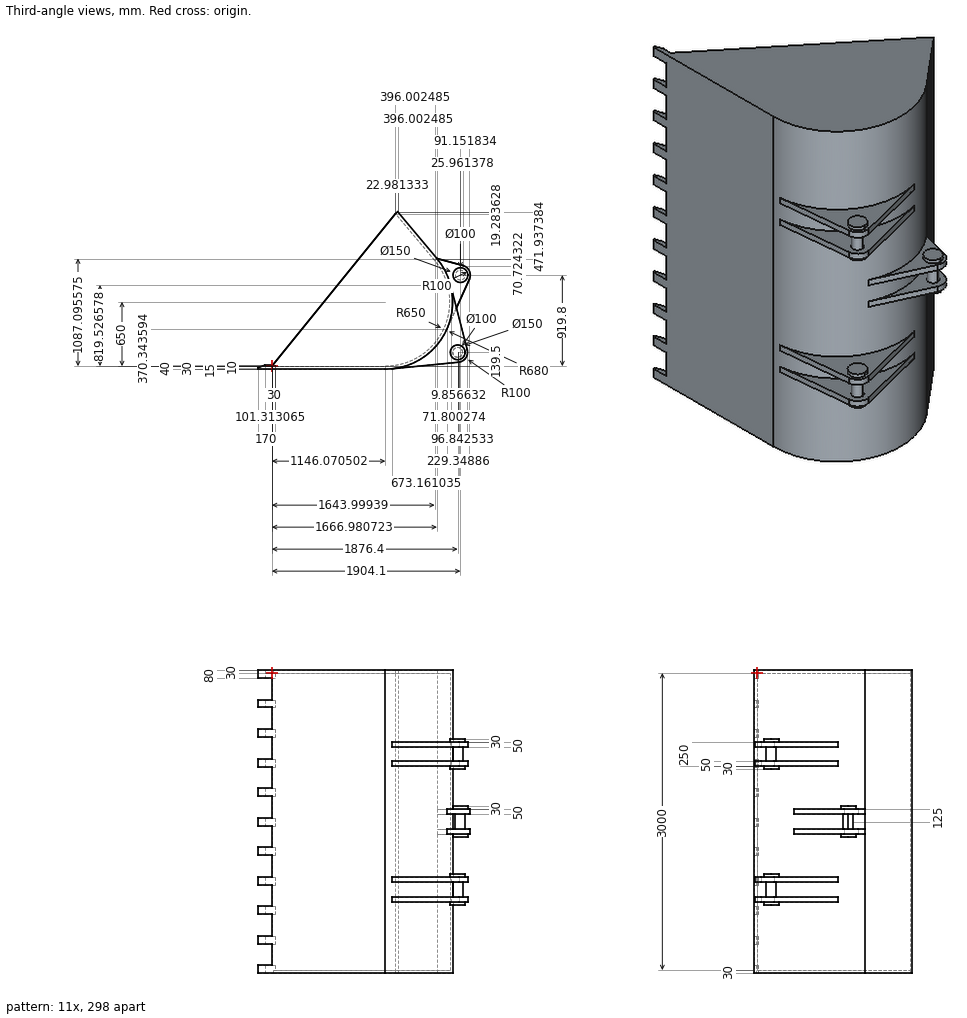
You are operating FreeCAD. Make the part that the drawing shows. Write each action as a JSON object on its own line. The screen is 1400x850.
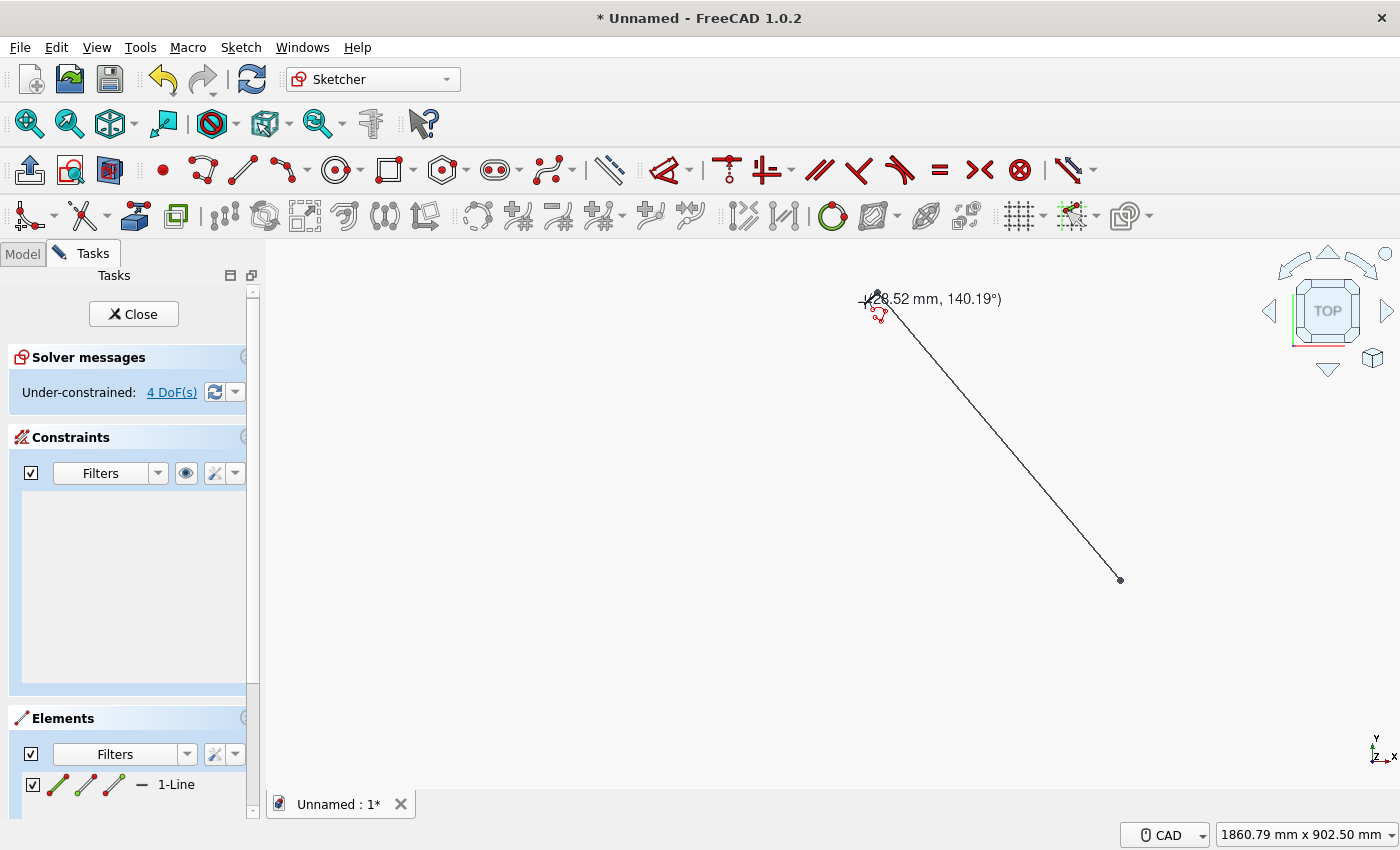
{"action": "left_click", "coordinate": [865, 302]}
{"action": "left_click", "coordinate": [1106, 590]}
{"action": "right_click", "coordinate": [1106, 590]}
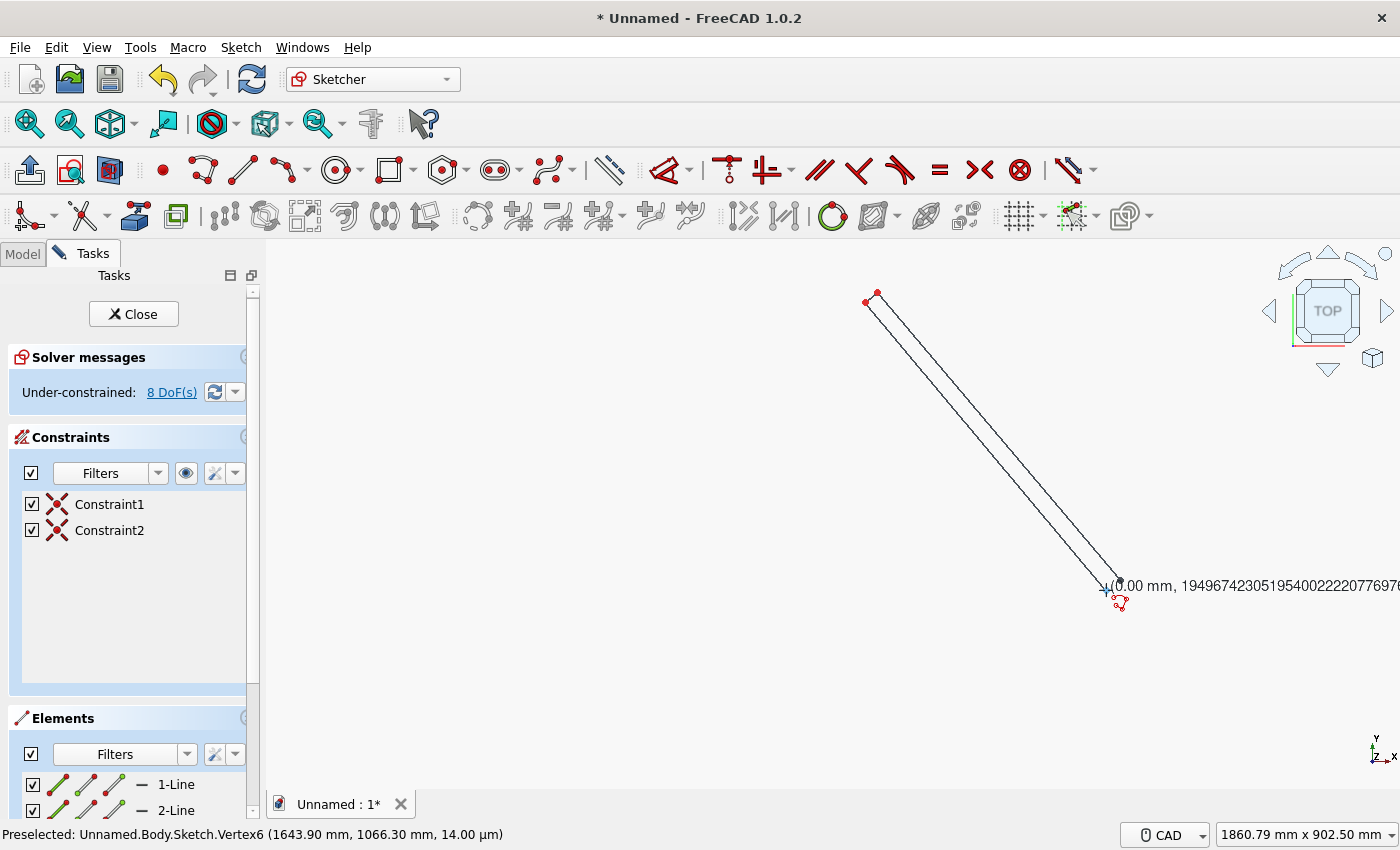
{"action": "scroll", "coordinate": [836, 362], "scroll_direction": "down", "scroll_amount": 5}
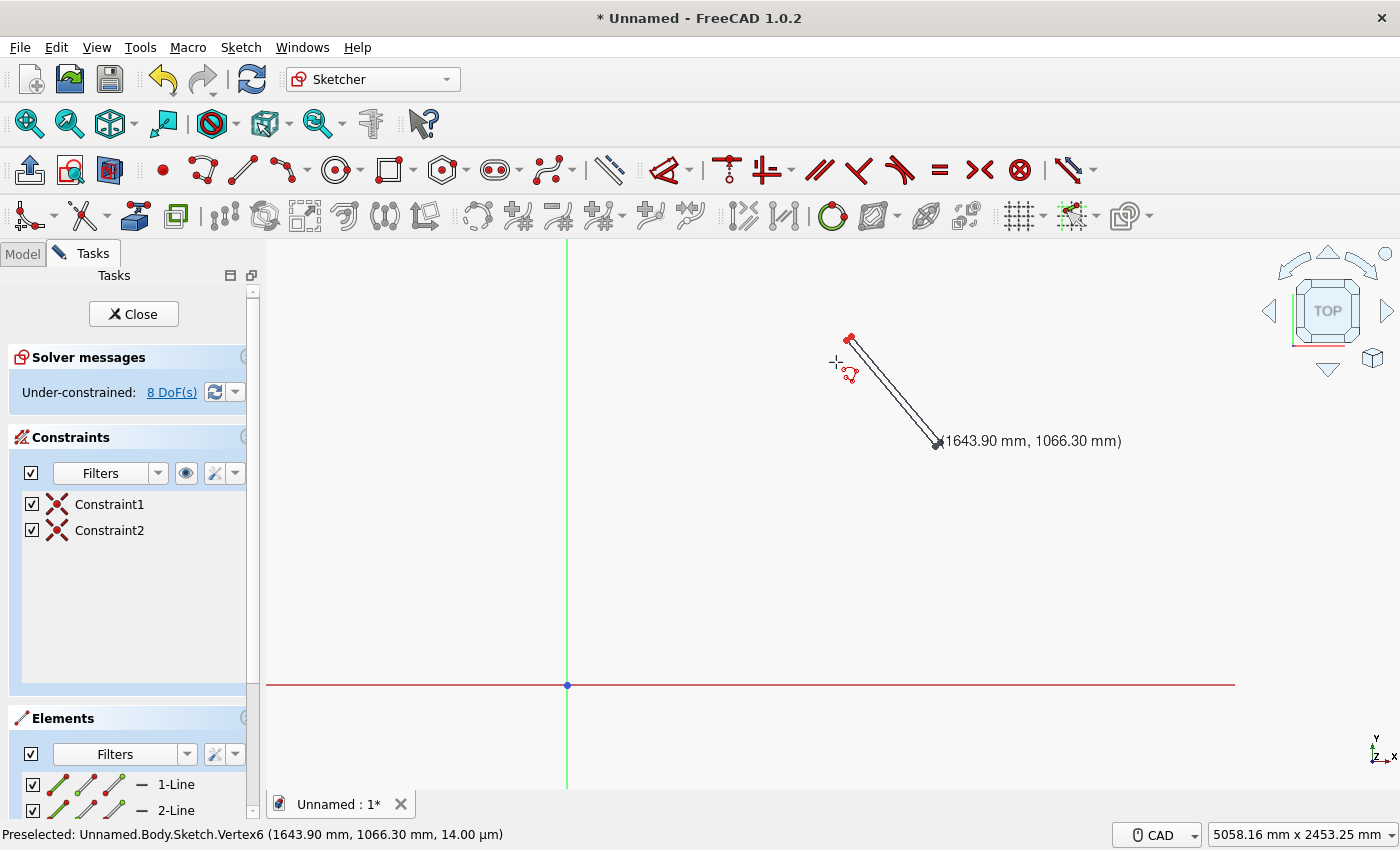
{"action": "left_click", "coordinate": [824, 685]}
{"action": "left_click", "coordinate": [567, 685]}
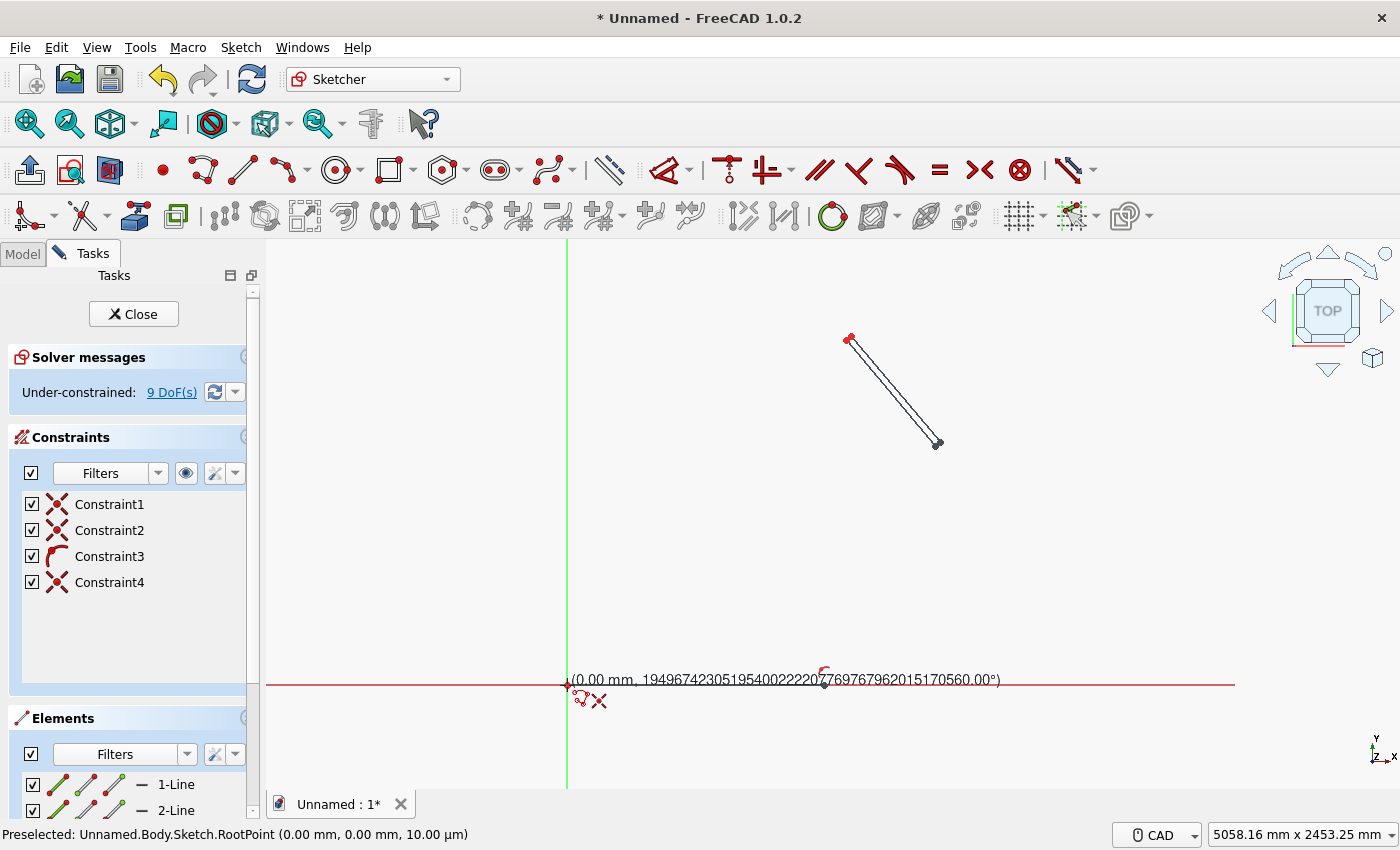
{"action": "scroll", "coordinate": [567, 692], "scroll_direction": "up", "scroll_amount": 5}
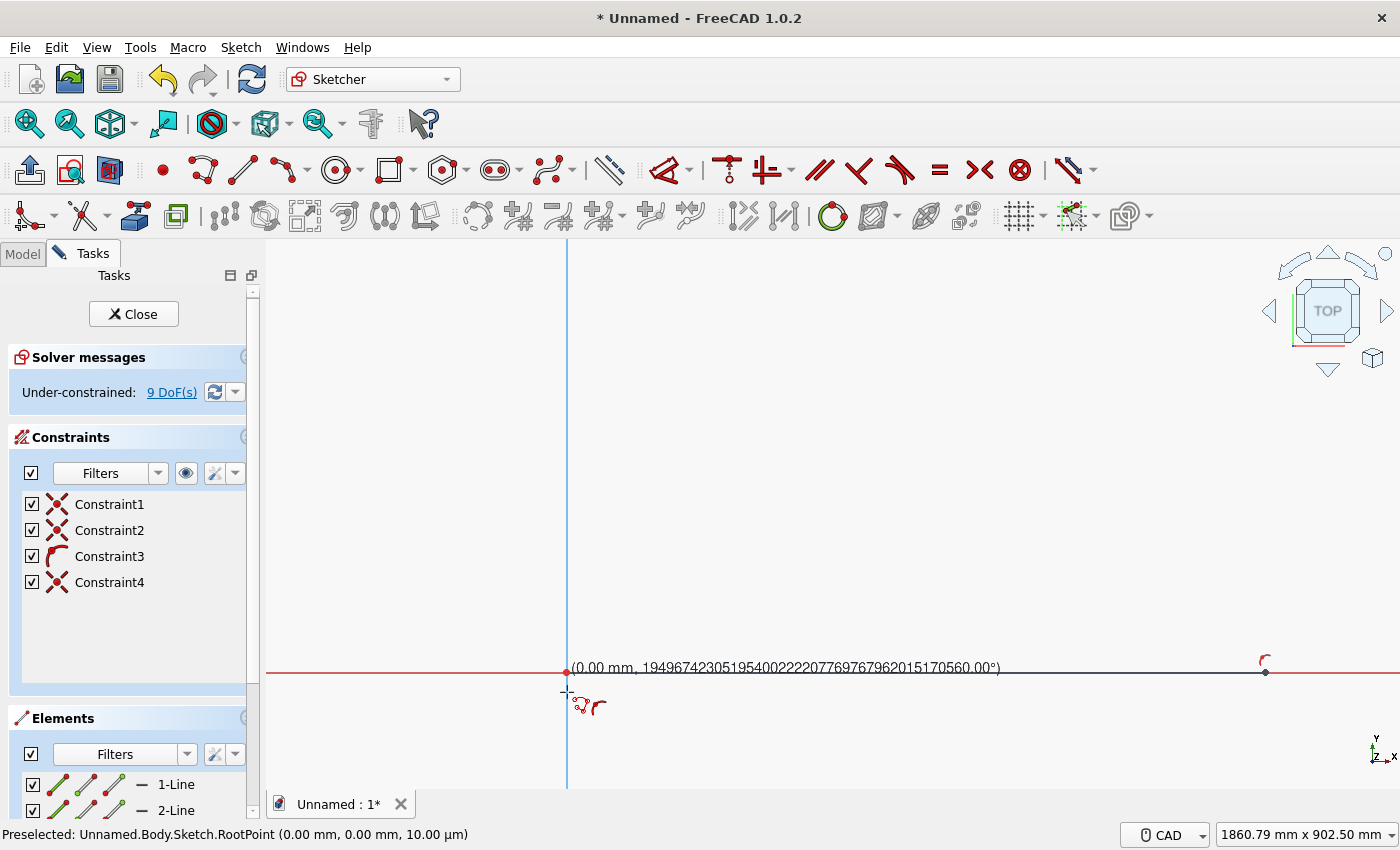
{"action": "left_click", "coordinate": [576, 691]}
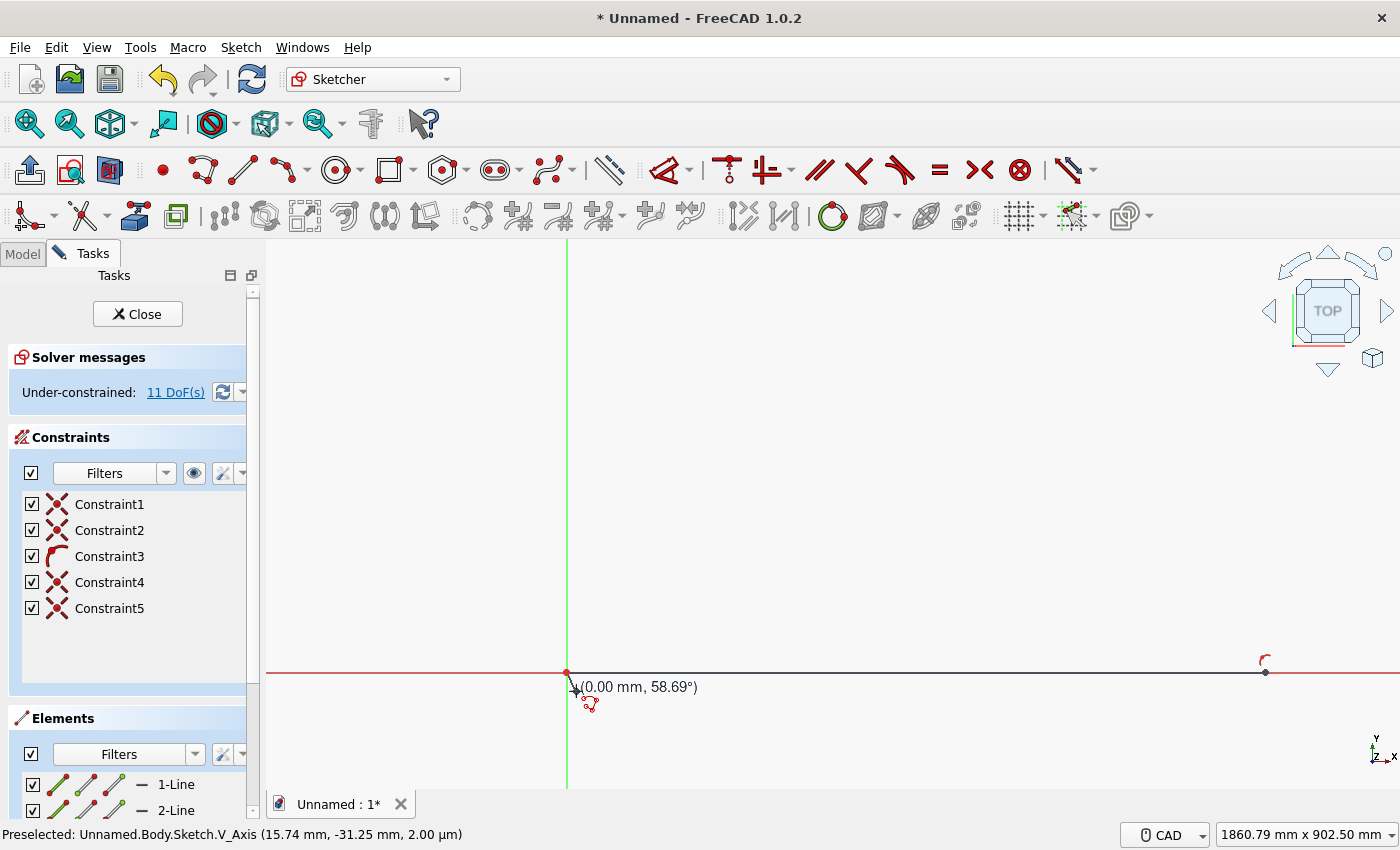
{"action": "scroll", "coordinate": [567, 693], "scroll_direction": "down", "scroll_amount": 5}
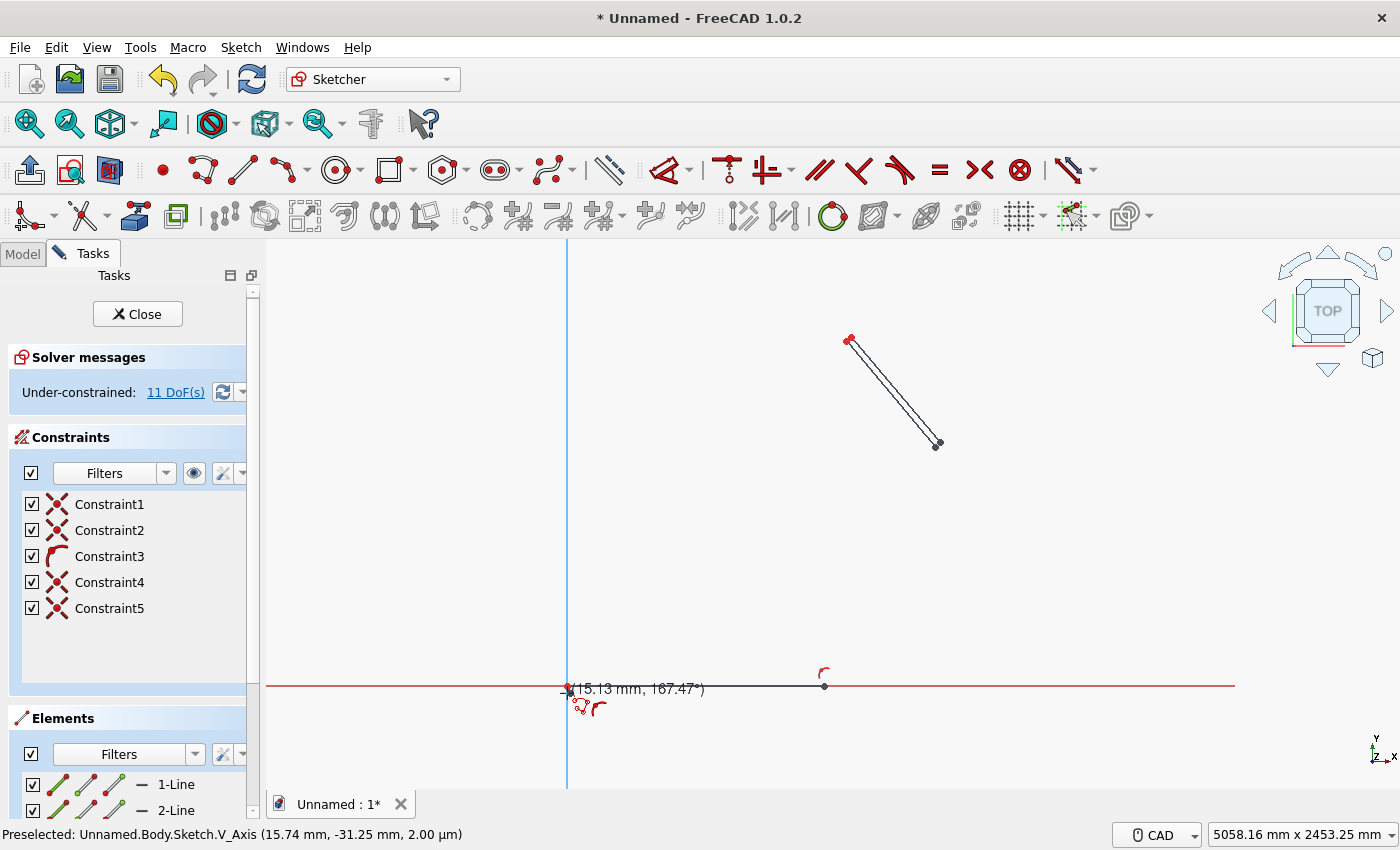
{"action": "scroll", "coordinate": [824, 693], "scroll_direction": "up", "scroll_amount": 5}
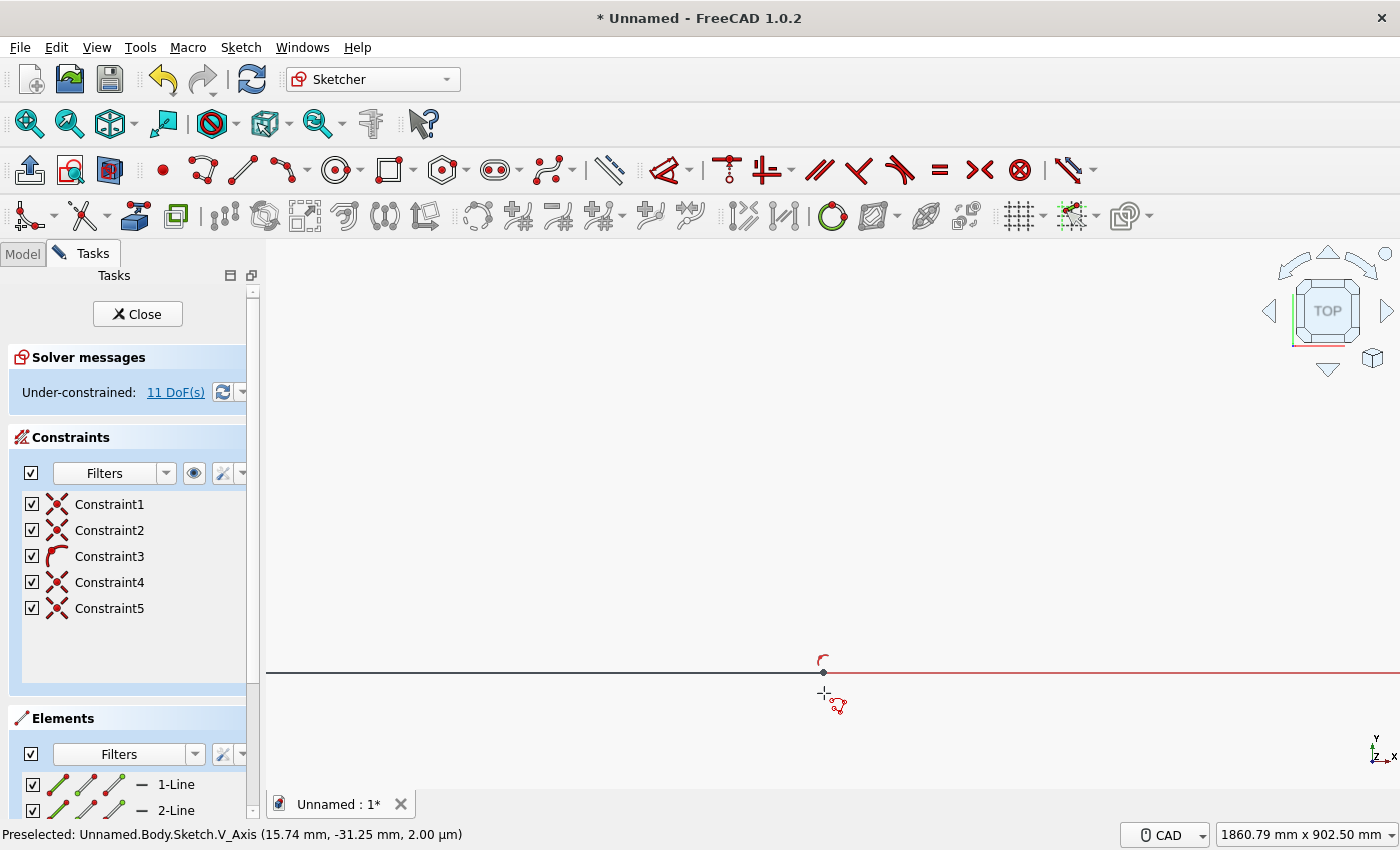
{"action": "left_click", "coordinate": [823, 691]}
{"action": "right_click", "coordinate": [823, 691]}